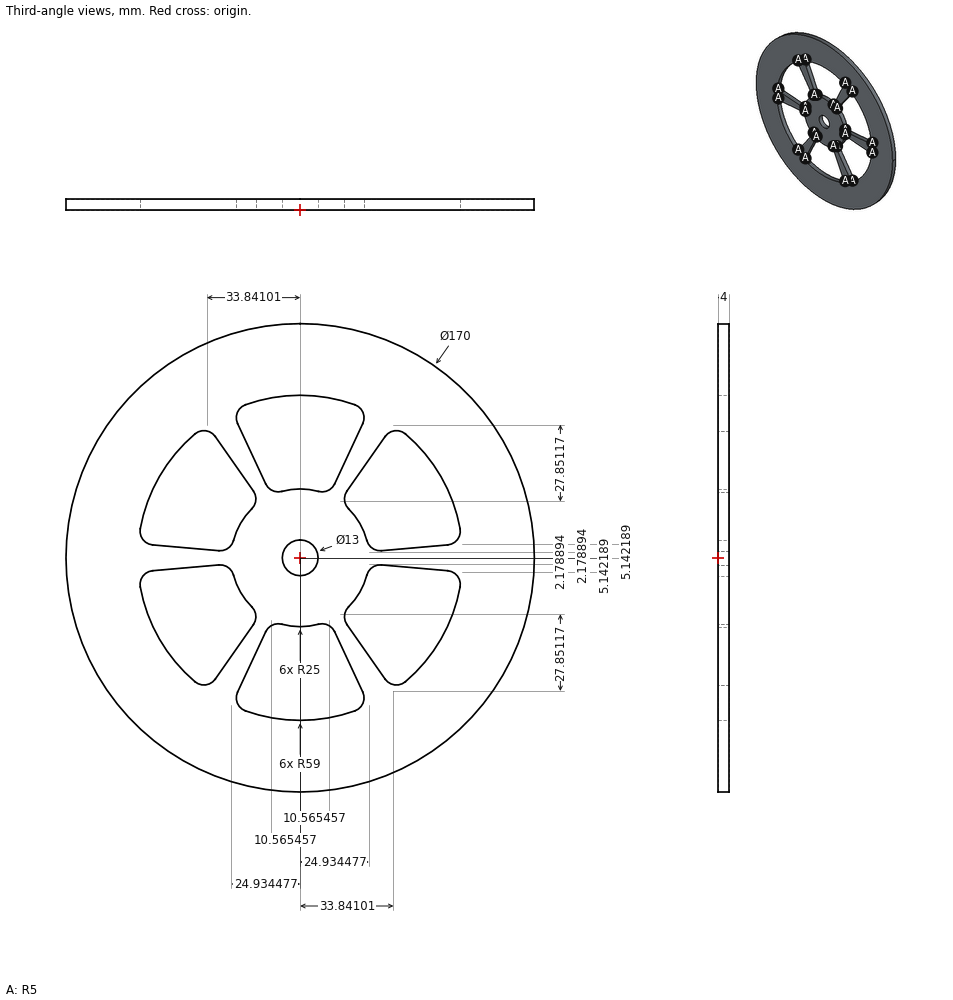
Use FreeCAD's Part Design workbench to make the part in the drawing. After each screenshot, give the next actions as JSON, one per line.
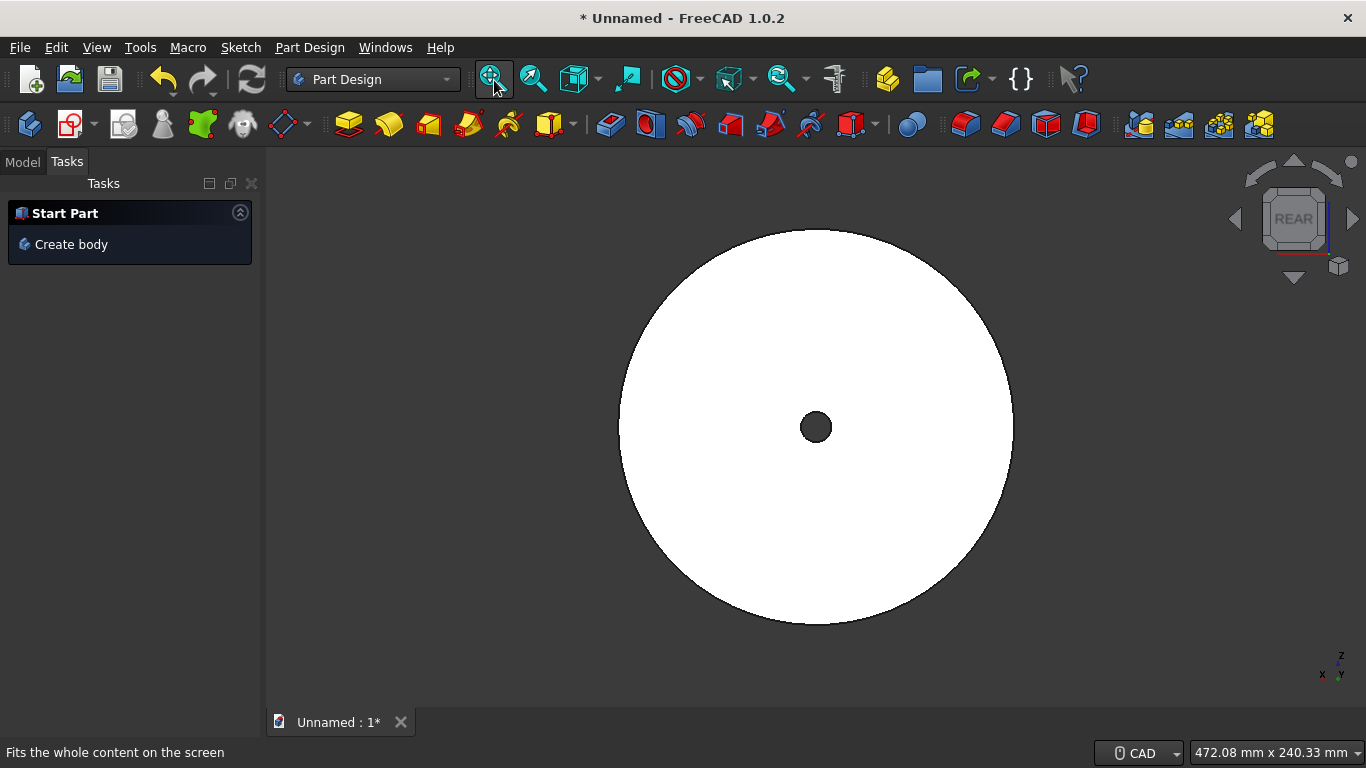
{"action": "left_click", "coordinate": [816, 539]}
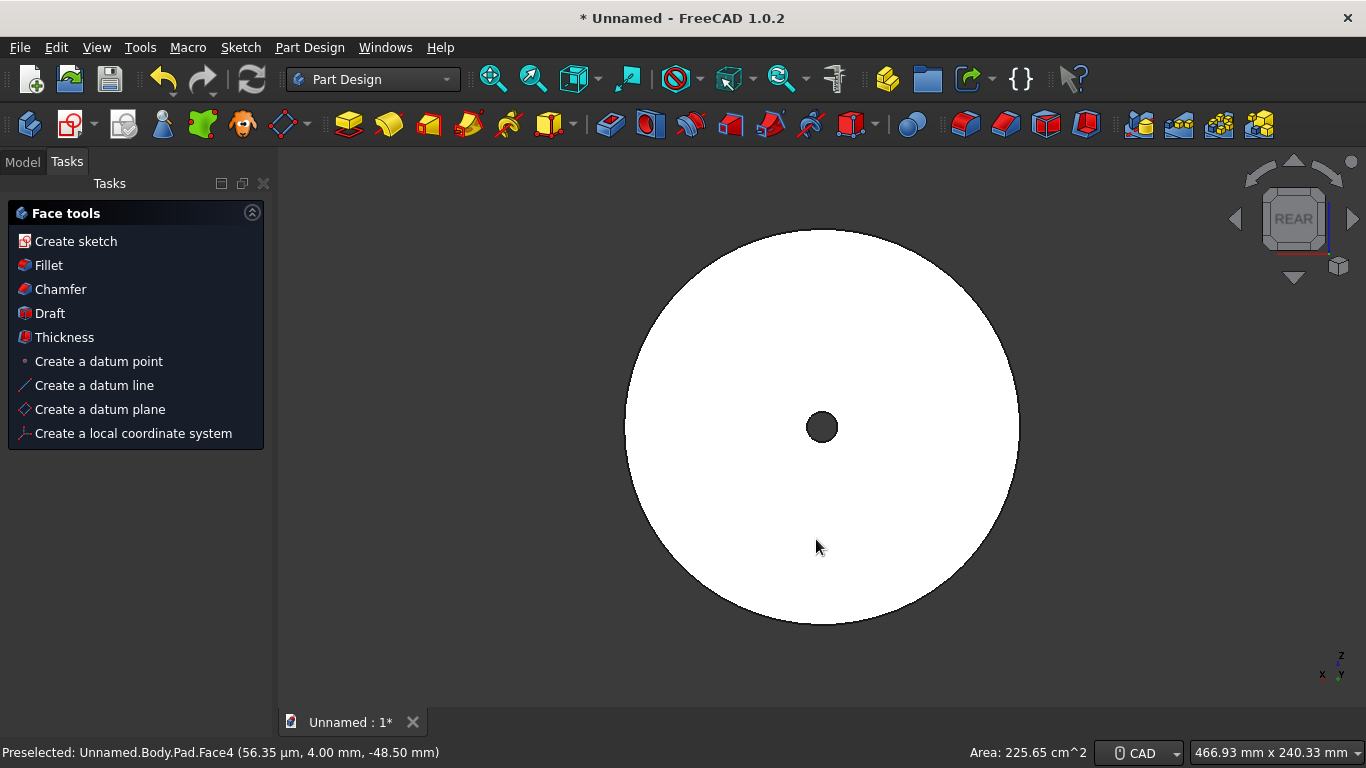
{"action": "left_click", "coordinate": [70, 124]}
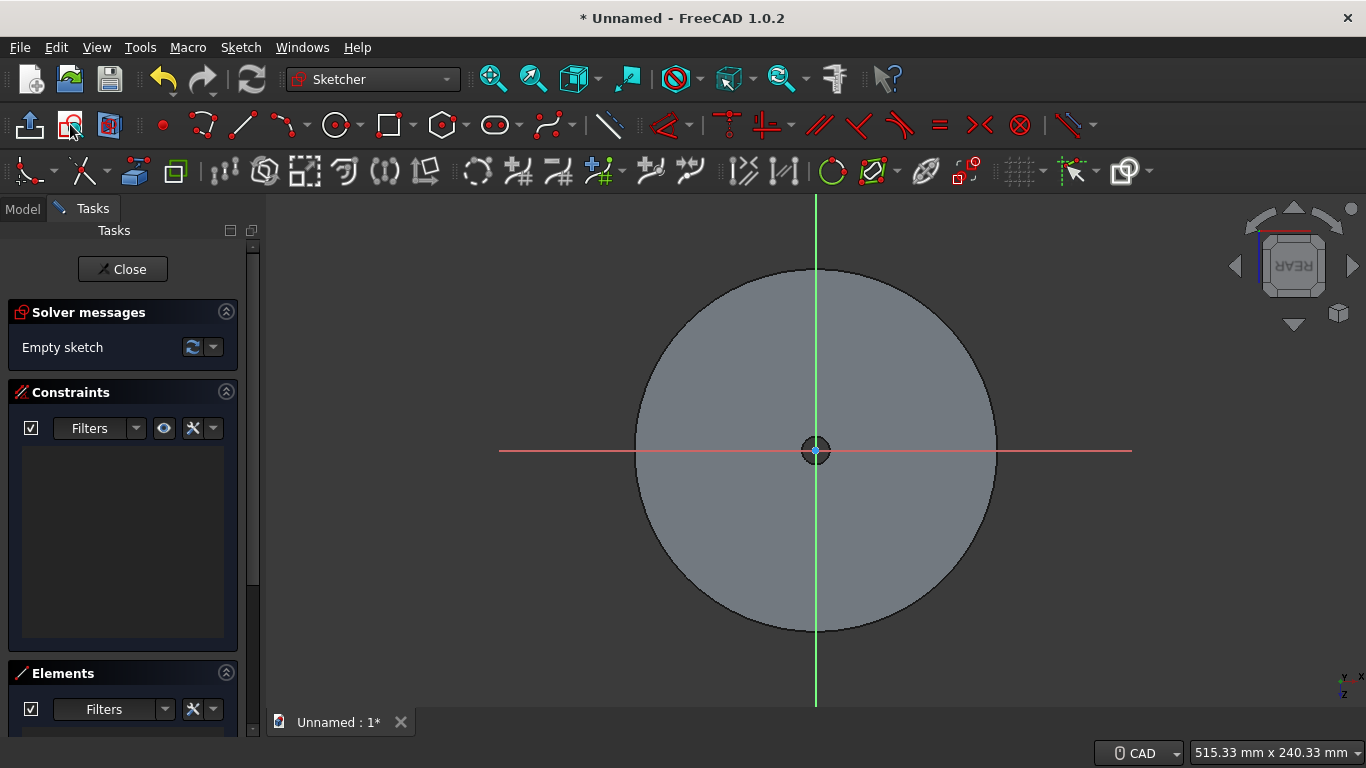
{"action": "left_click", "coordinate": [244, 126]}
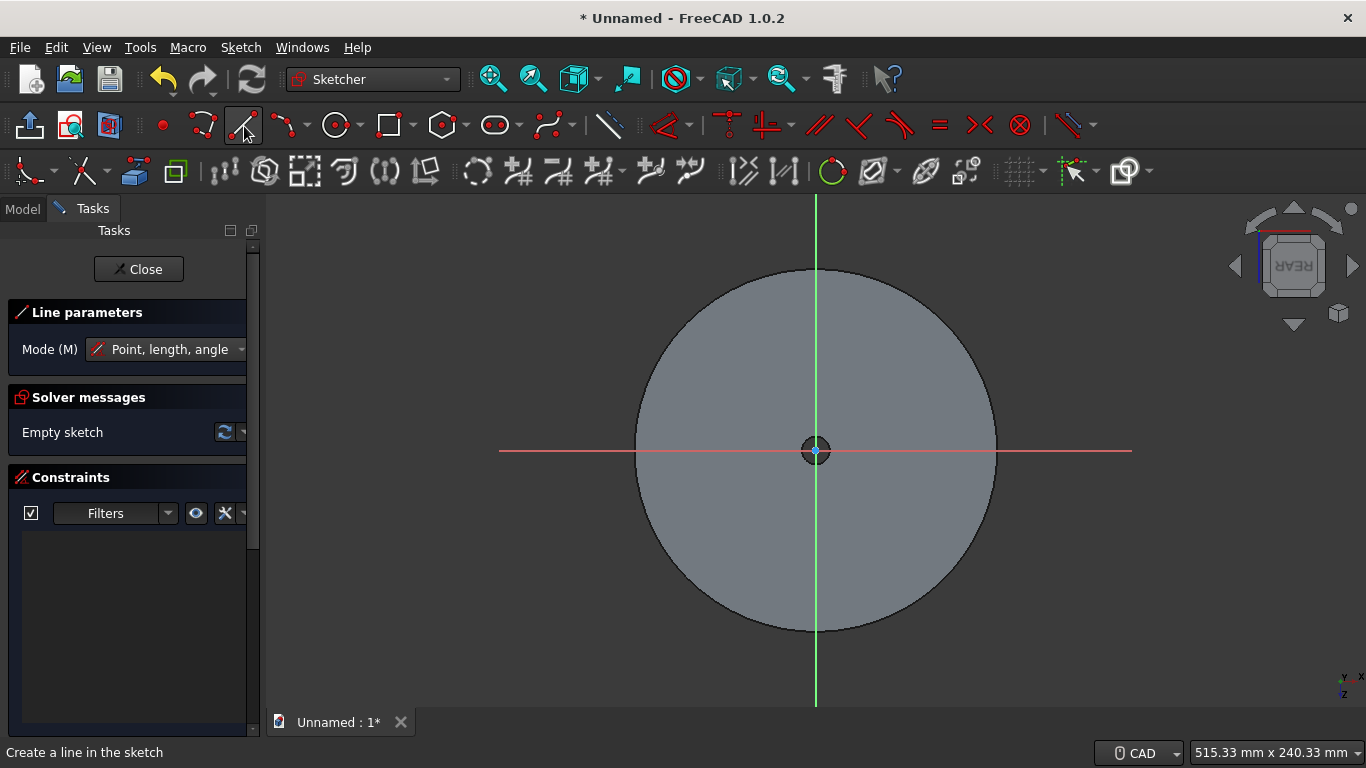
{"action": "left_click", "coordinate": [838, 402]}
{"action": "left_click", "coordinate": [869, 336]}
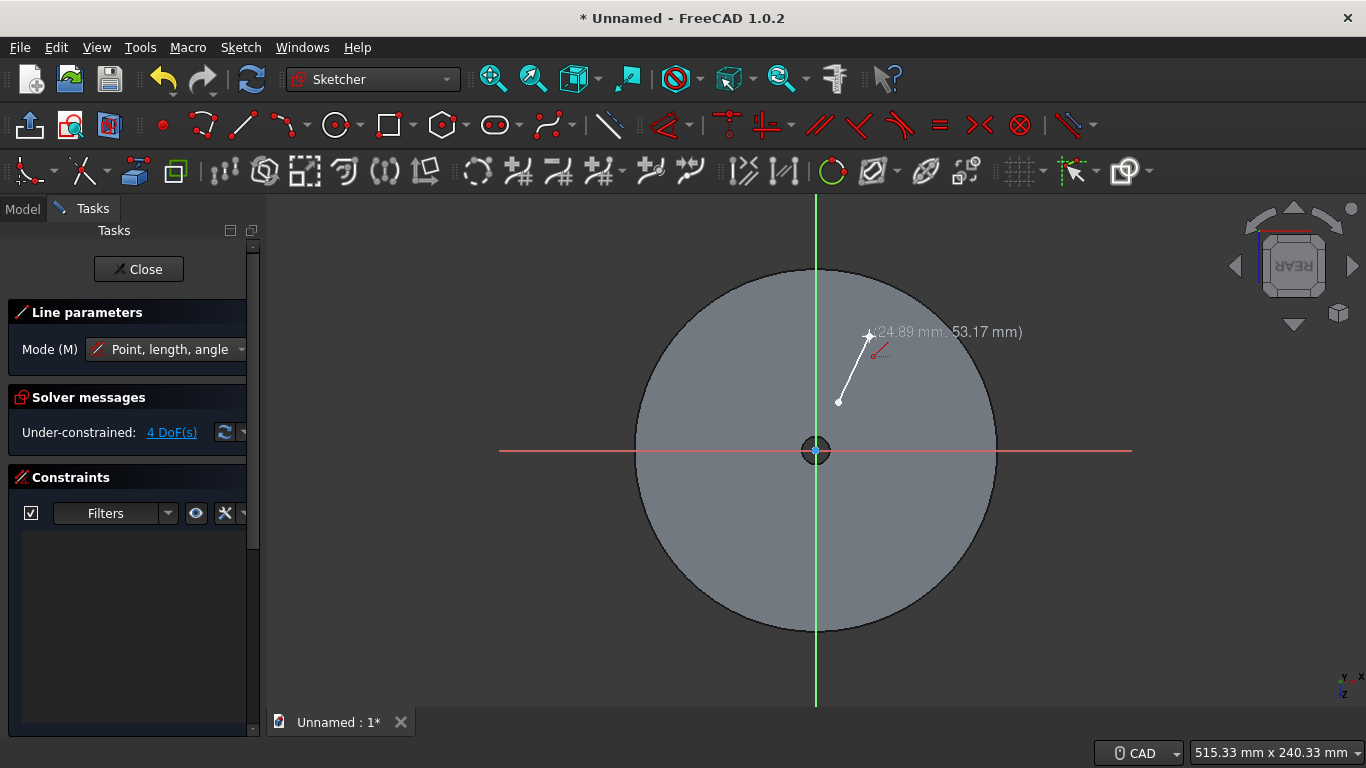
{"action": "left_click", "coordinate": [763, 336]}
{"action": "left_click", "coordinate": [793, 402]}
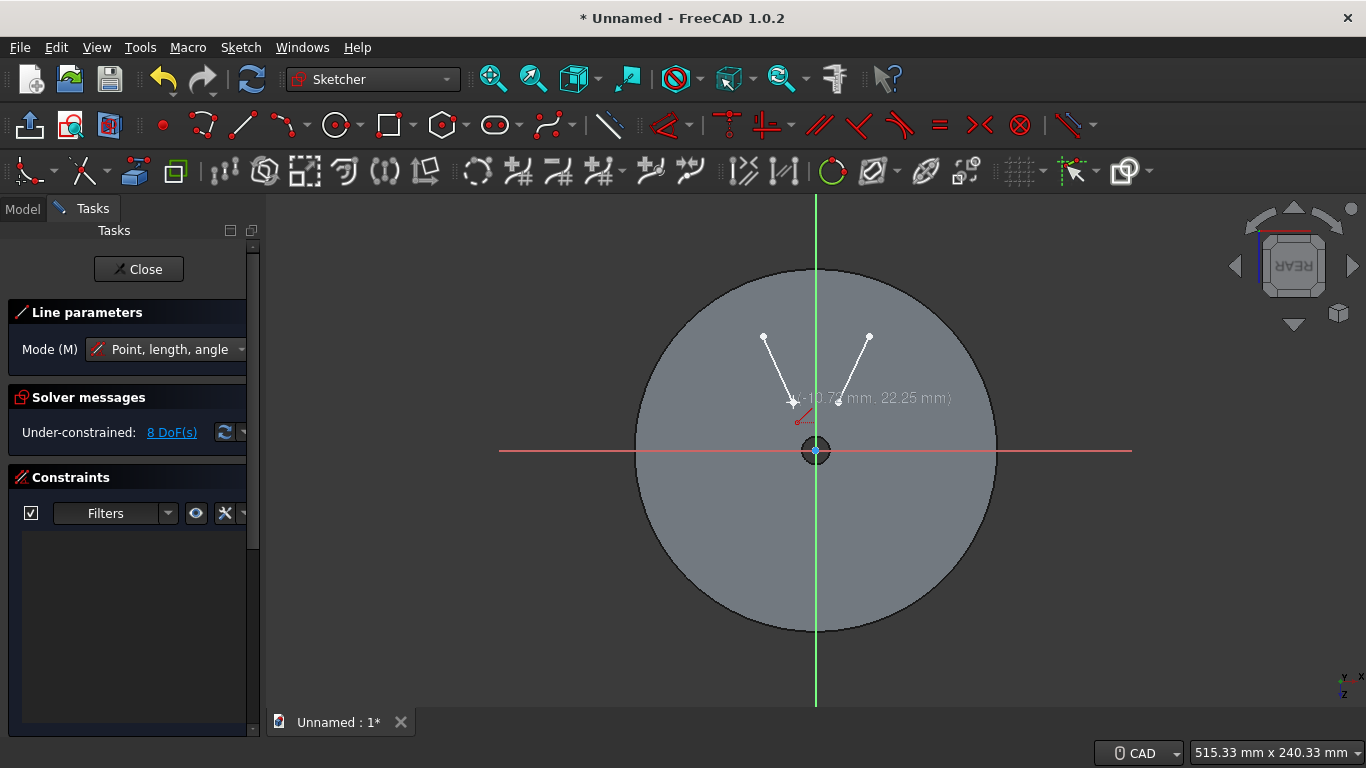
{"action": "left_click", "coordinate": [284, 126]}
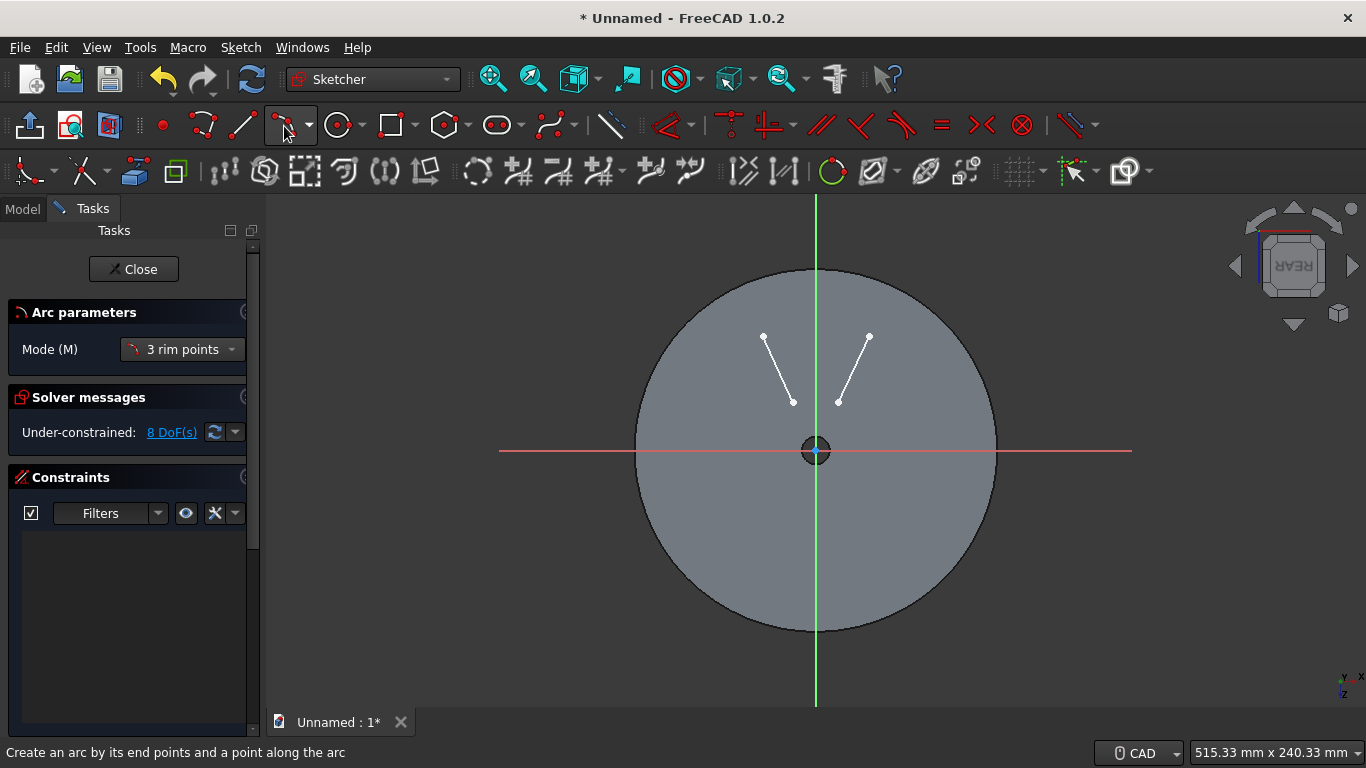
{"action": "left_click", "coordinate": [869, 337]}
{"action": "left_click", "coordinate": [763, 337]}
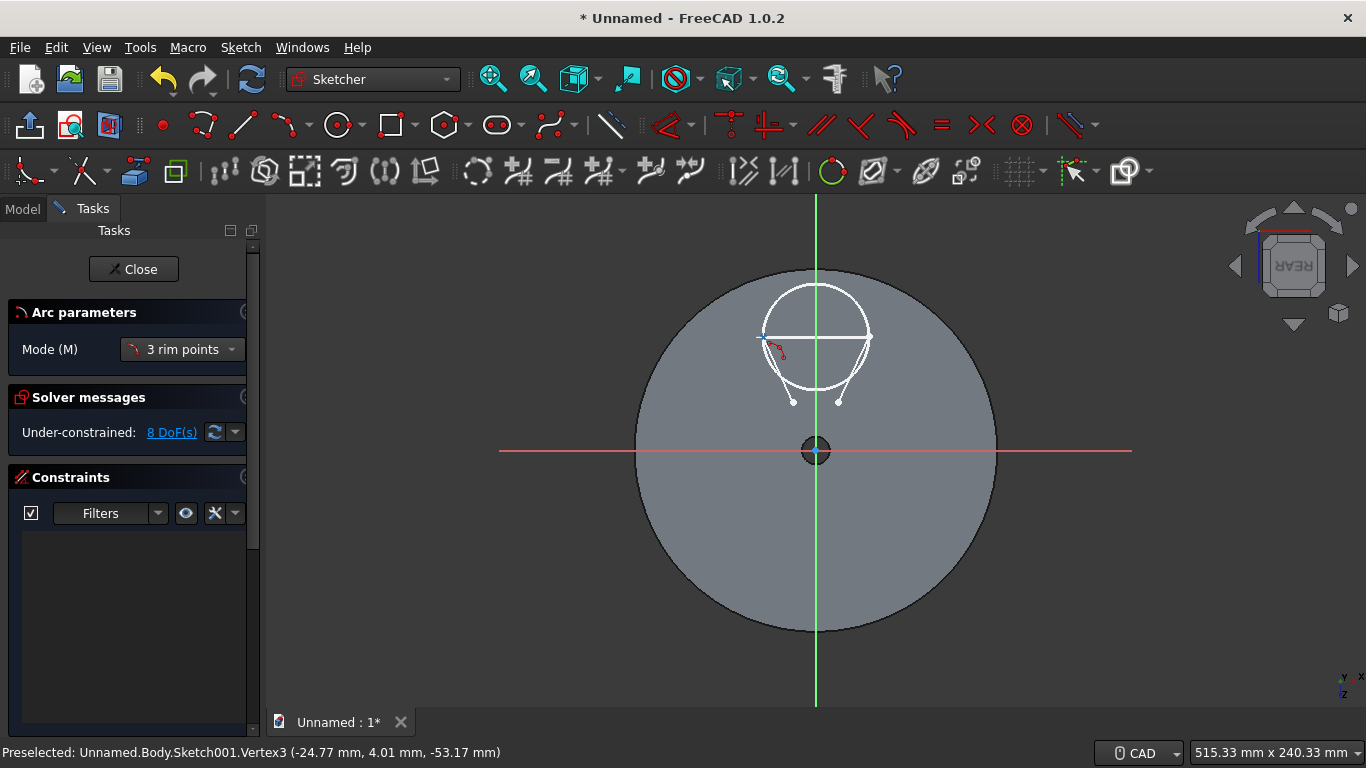
{"action": "scroll", "coordinate": [827, 325], "scroll_direction": "up", "scroll_amount": 2}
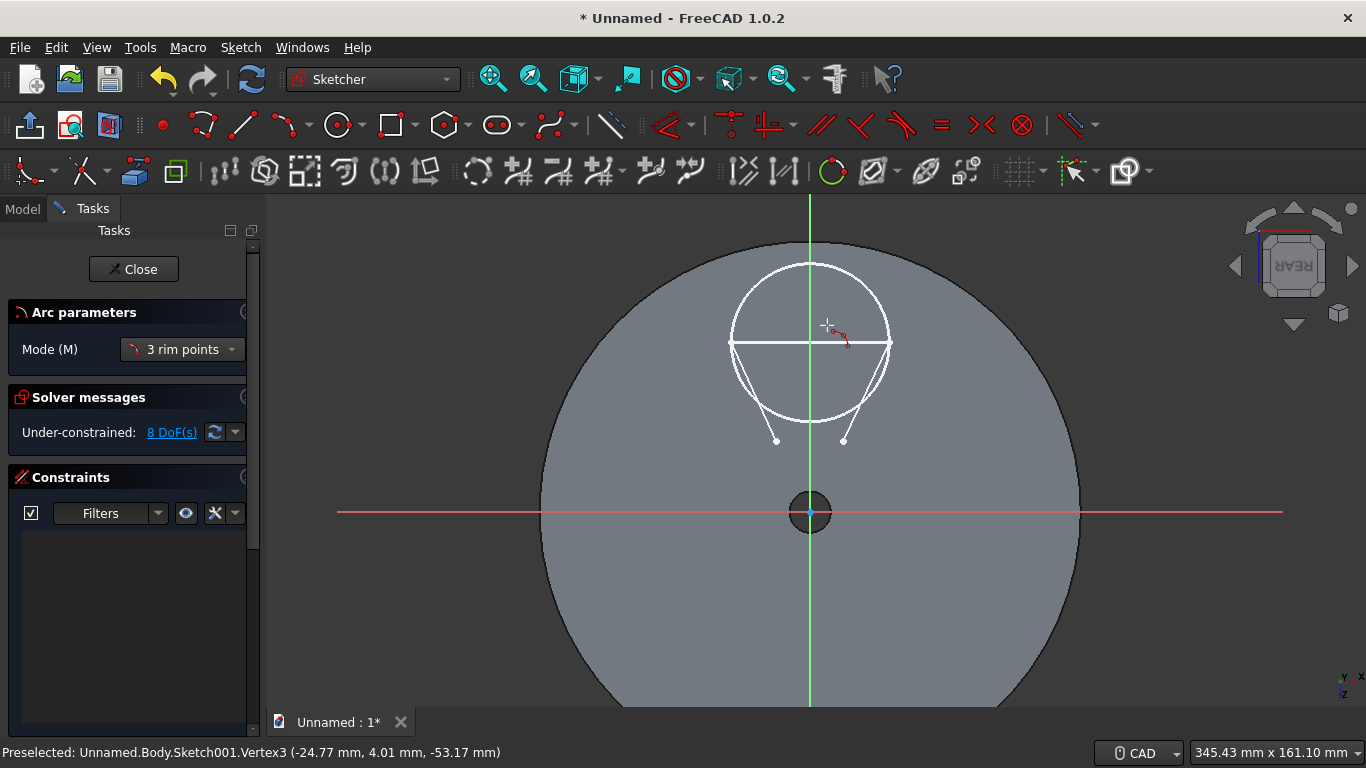
{"action": "left_click", "coordinate": [827, 325]}